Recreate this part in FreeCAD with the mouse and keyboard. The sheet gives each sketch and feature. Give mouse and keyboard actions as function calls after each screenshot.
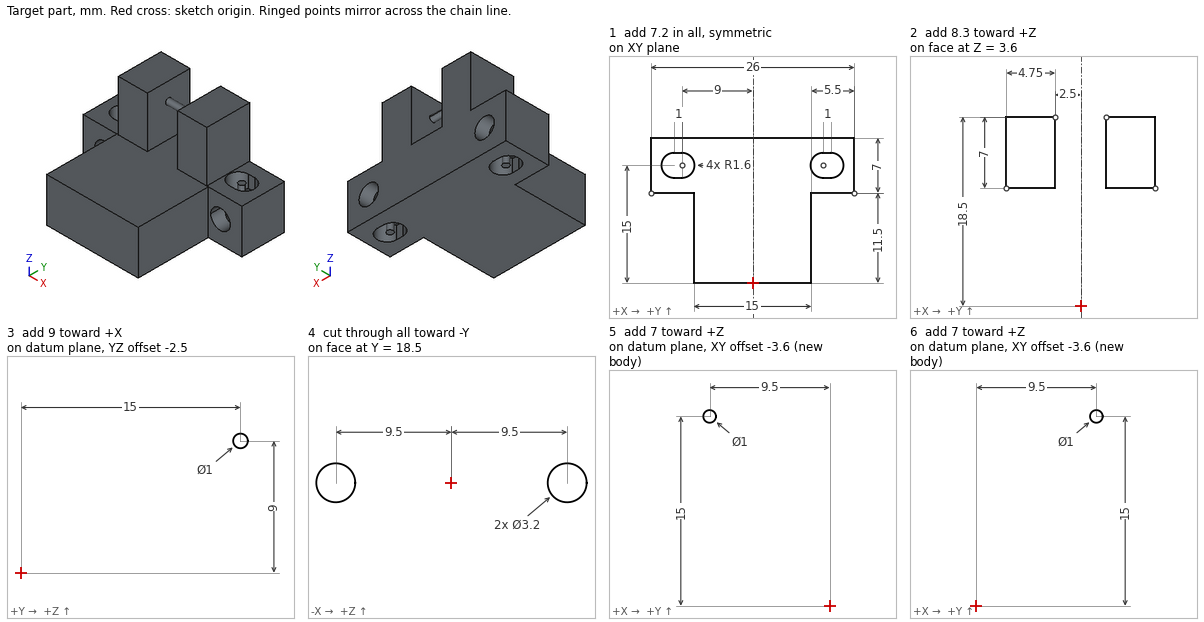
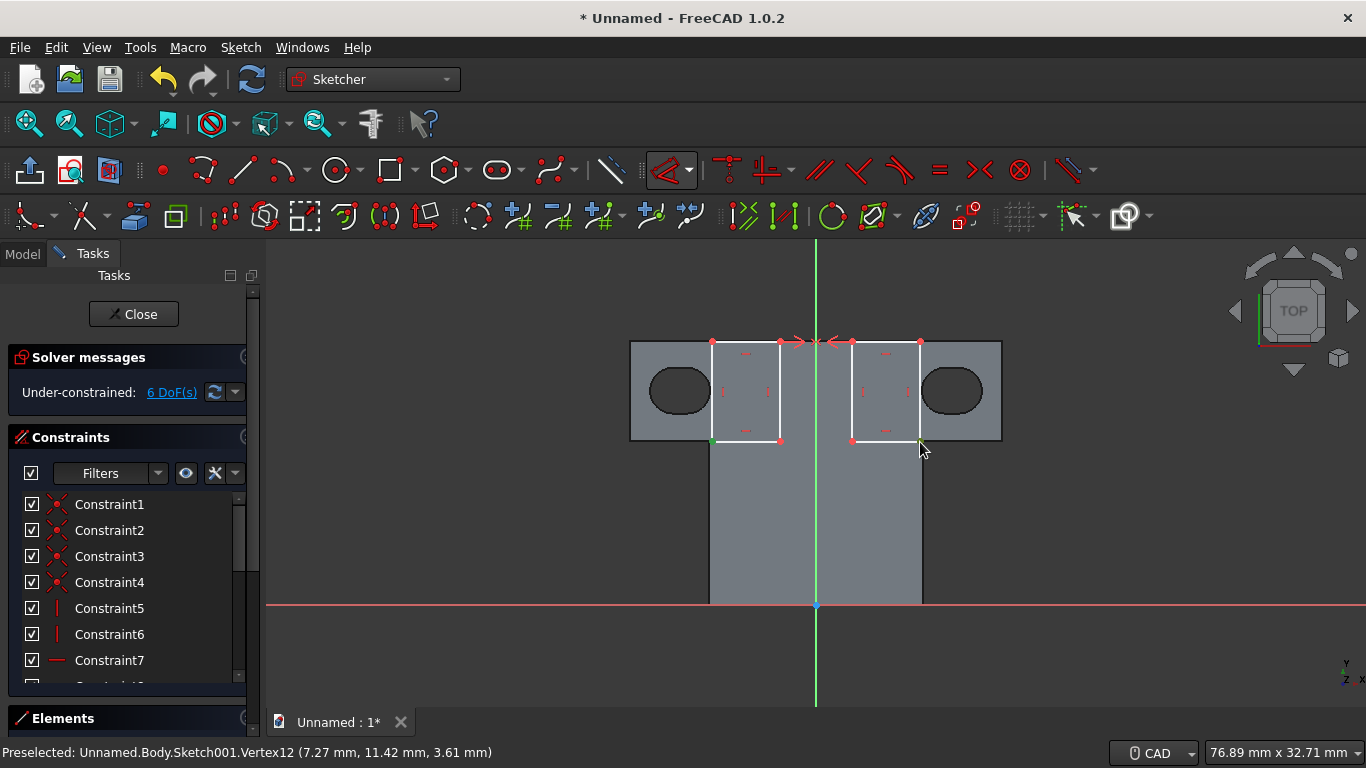
click(816, 650)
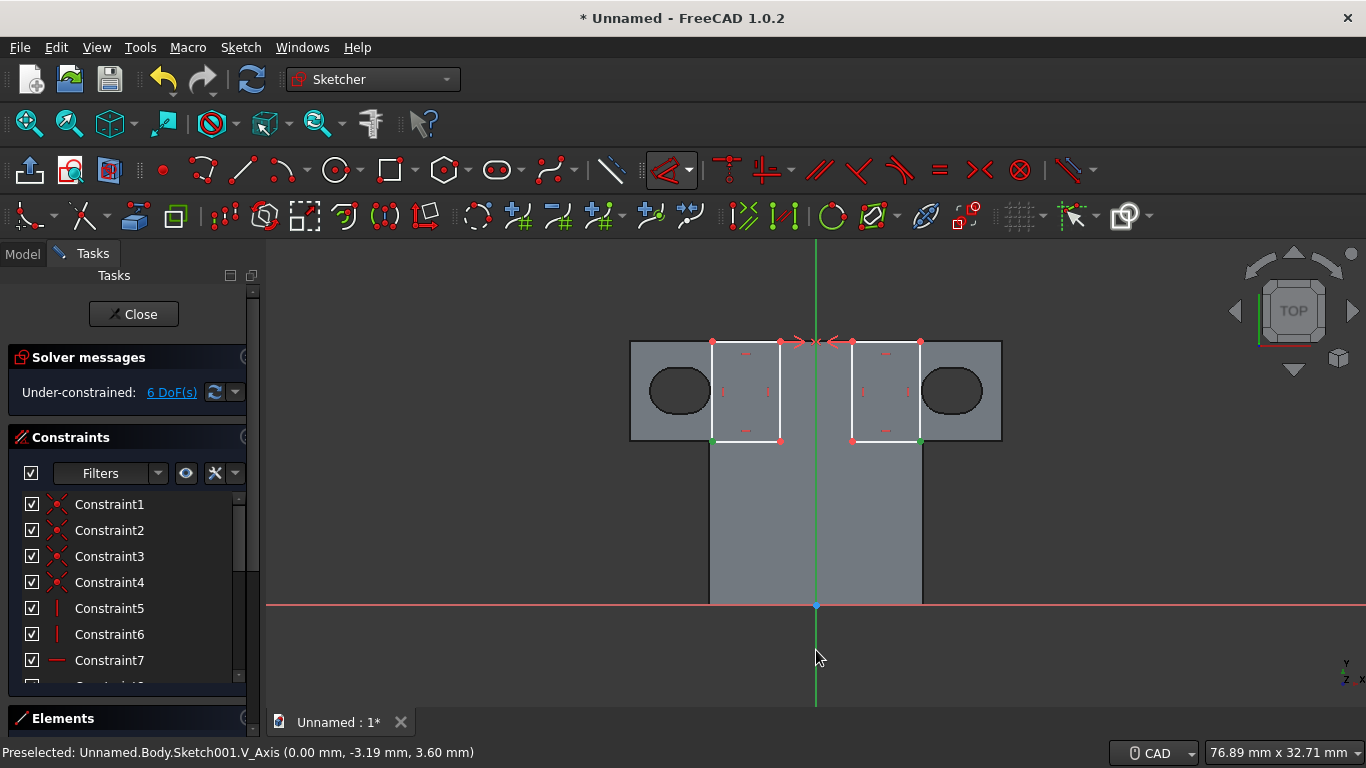
key(s)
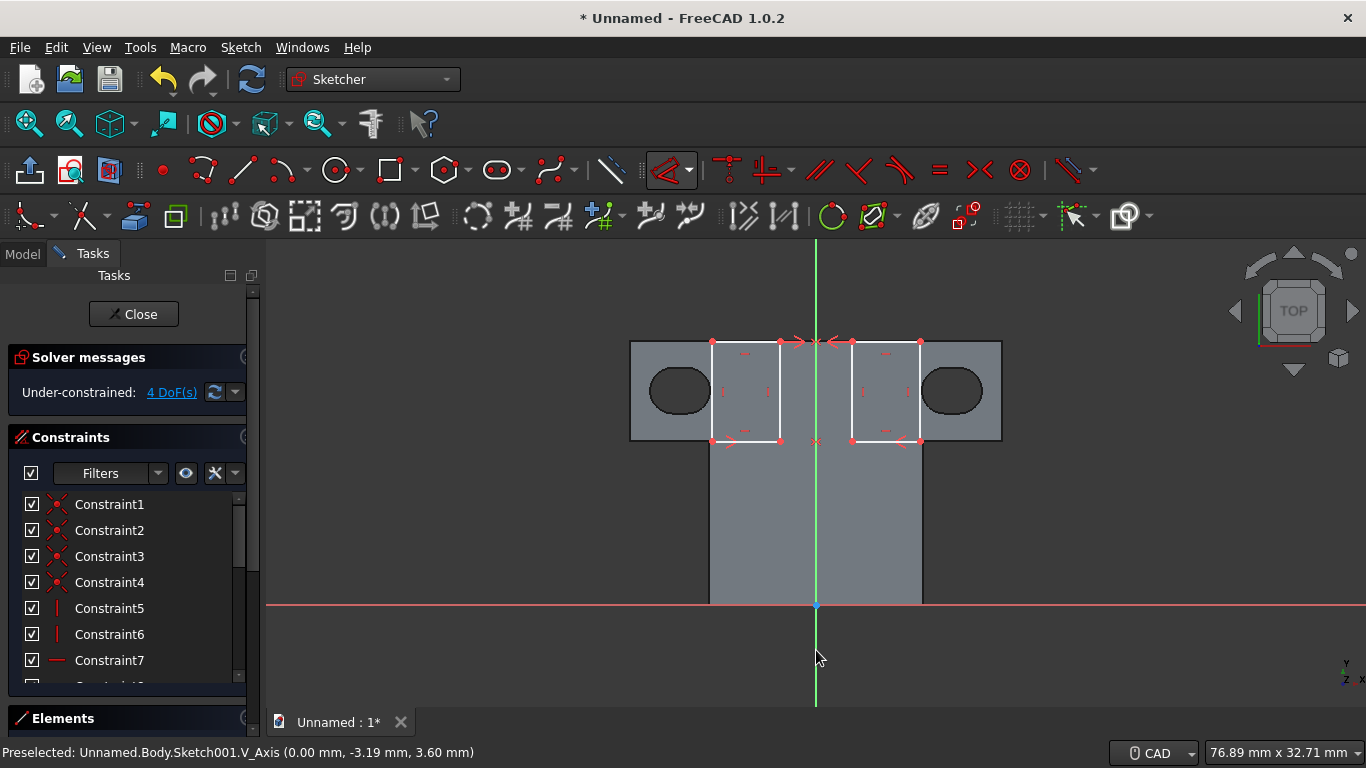
click(712, 372)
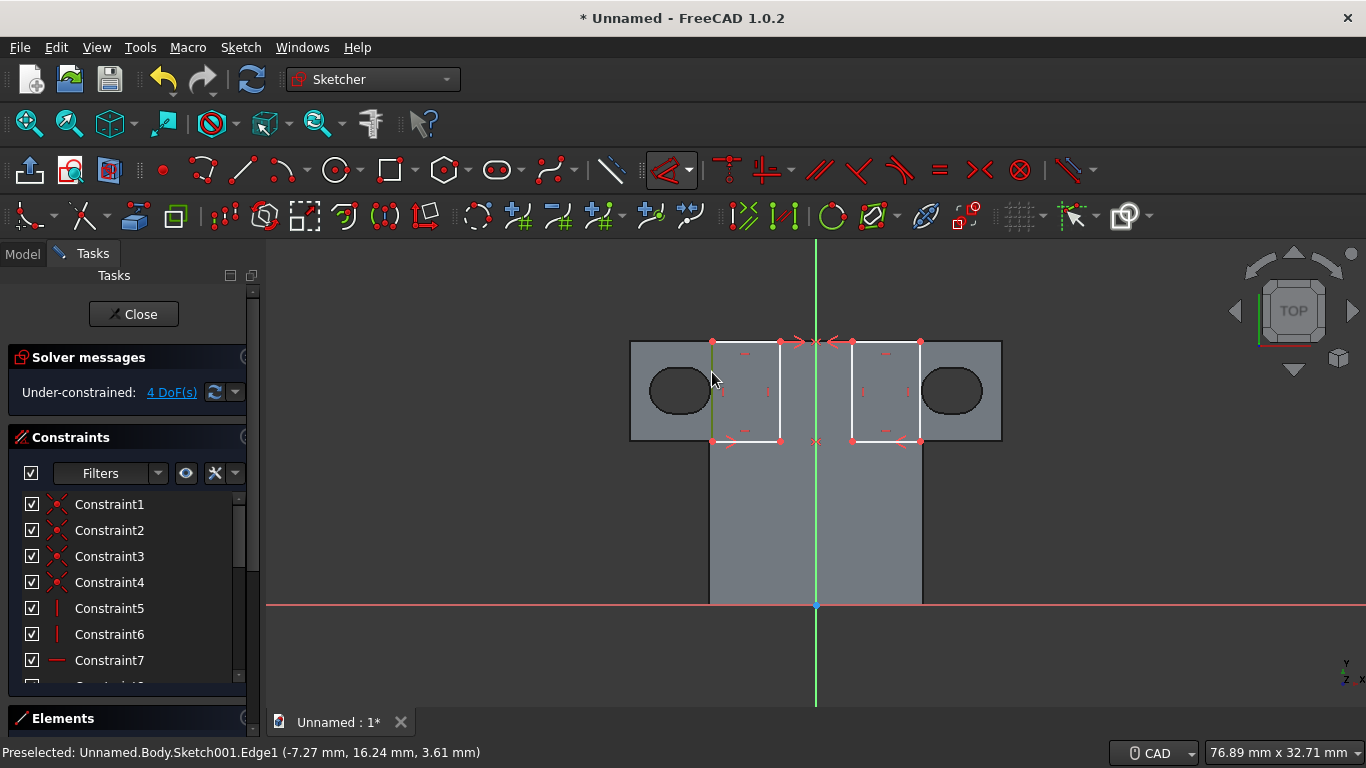
key(i)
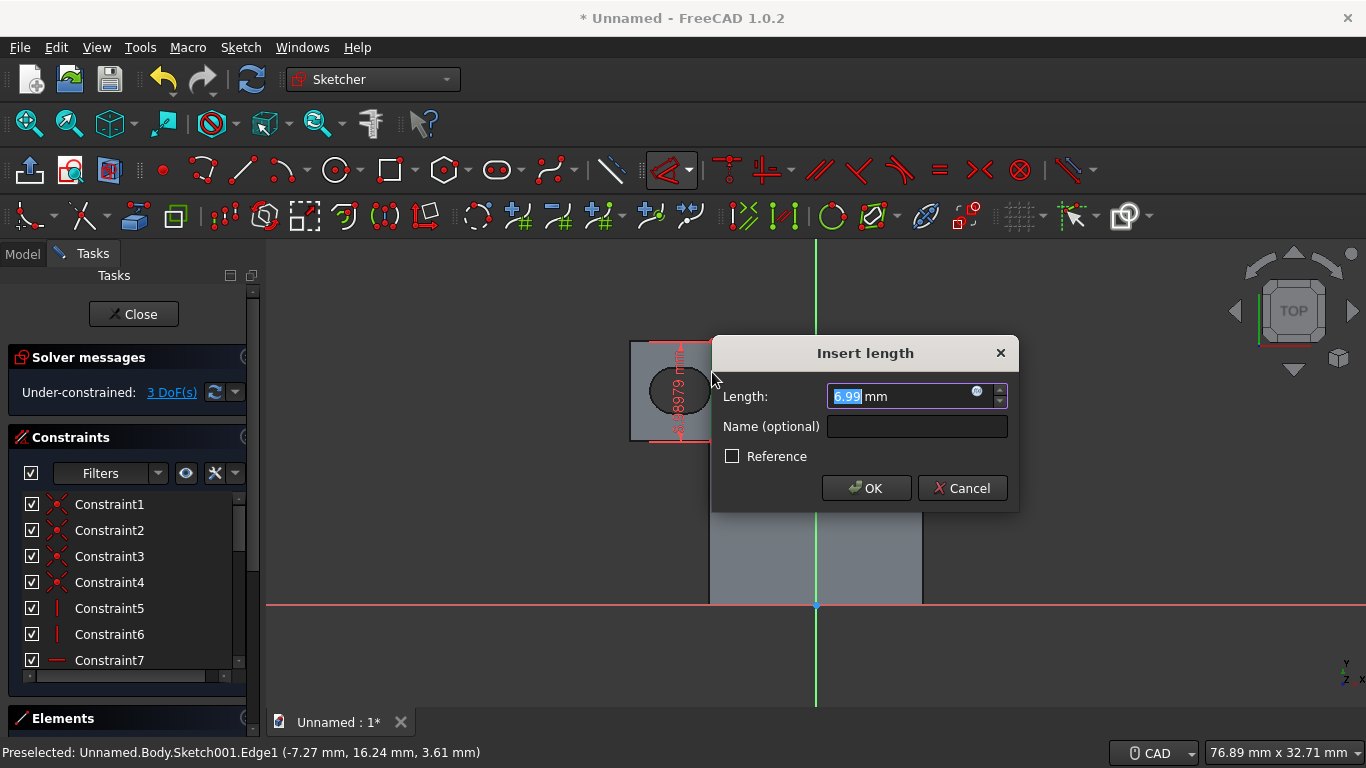
text(7)
key(Return)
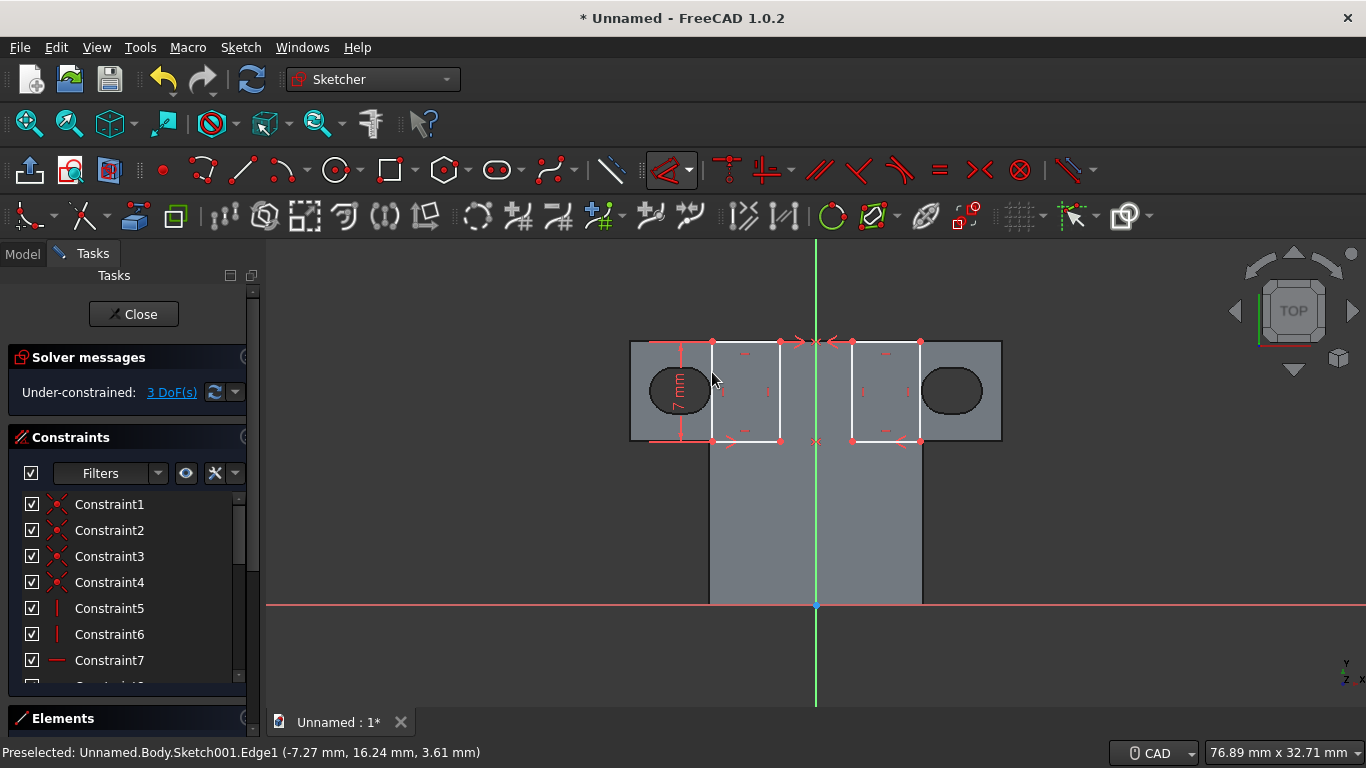
click(732, 442)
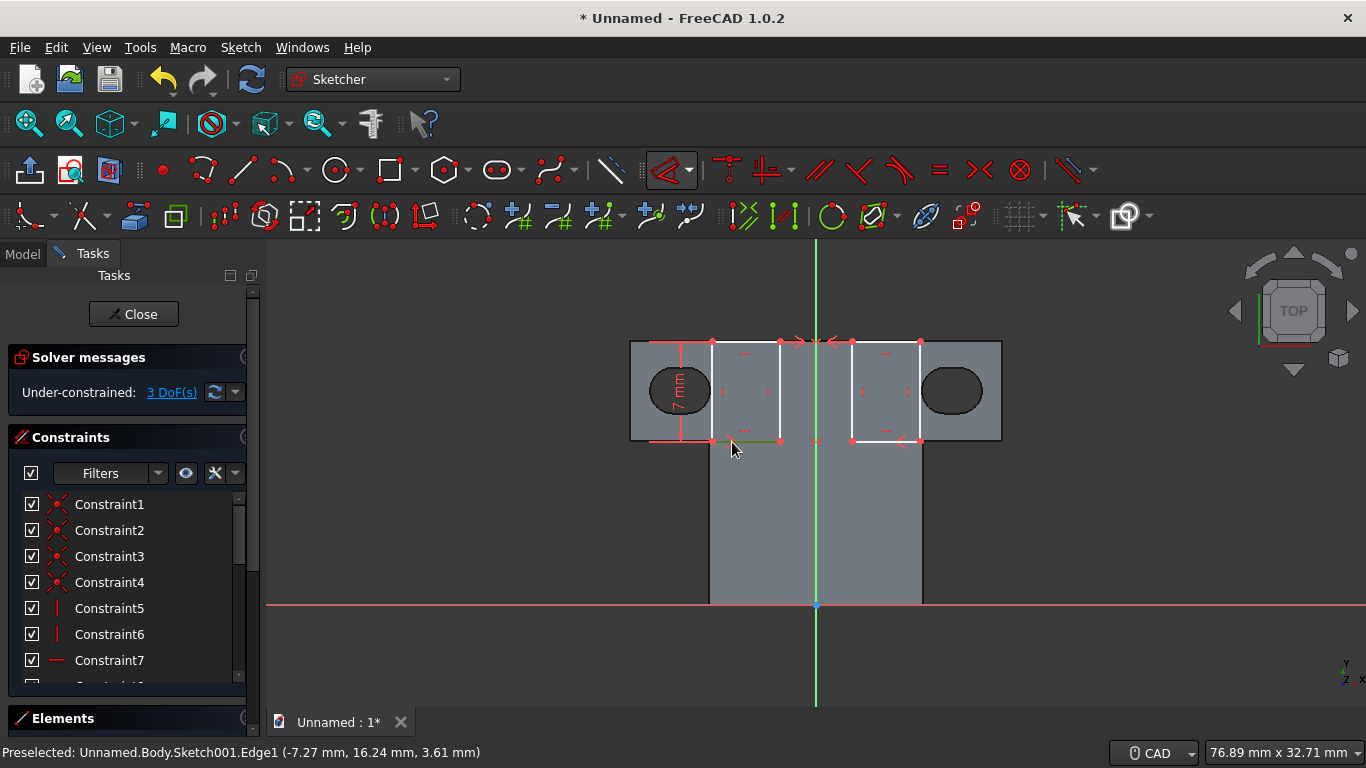
key(l)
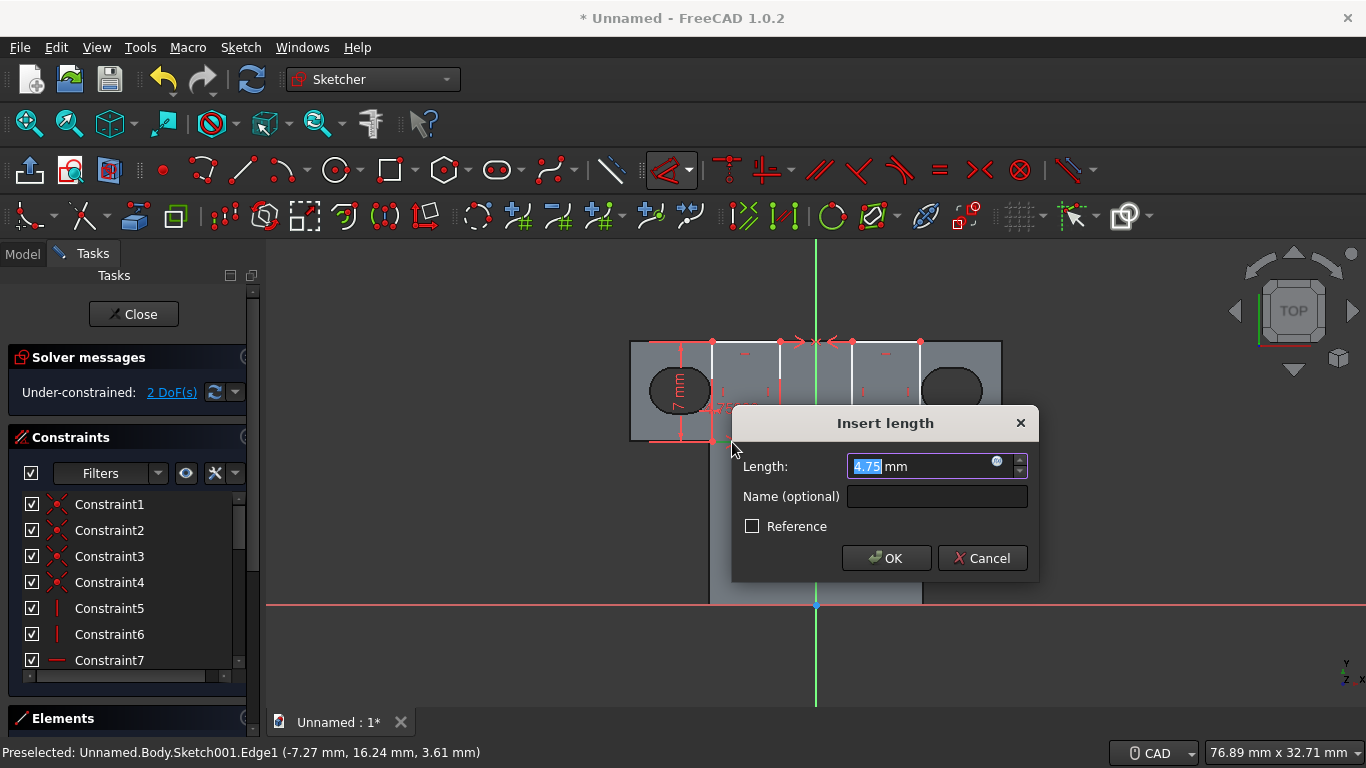
text(4.75)
key(Return)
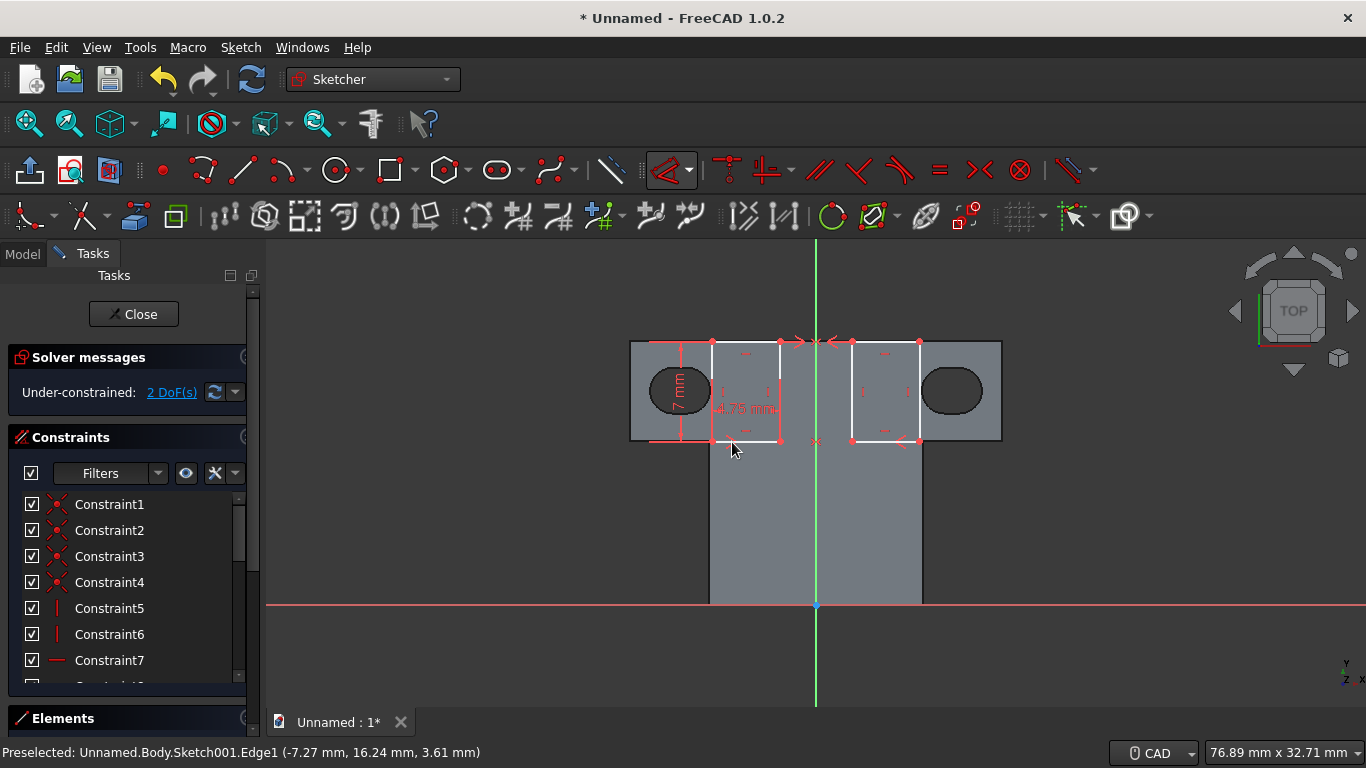
click(780, 442)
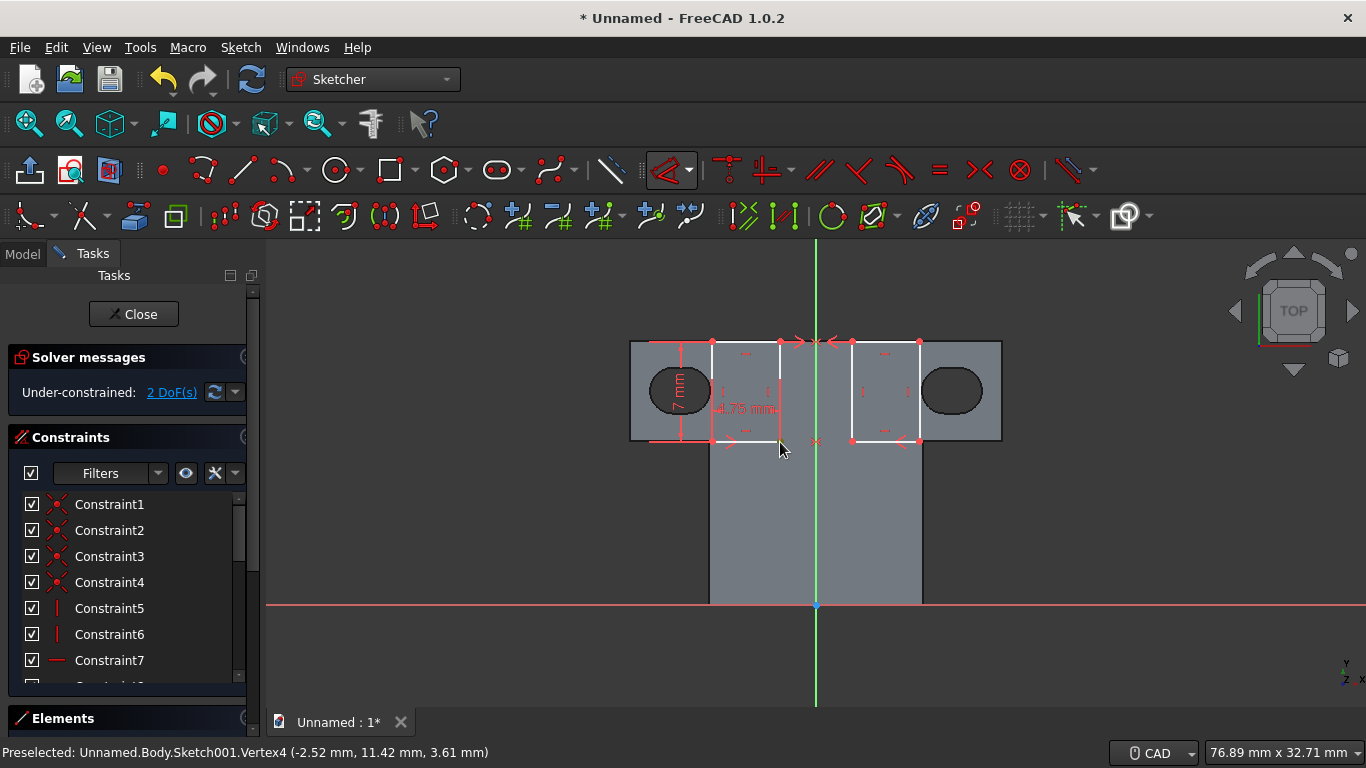
key(l)